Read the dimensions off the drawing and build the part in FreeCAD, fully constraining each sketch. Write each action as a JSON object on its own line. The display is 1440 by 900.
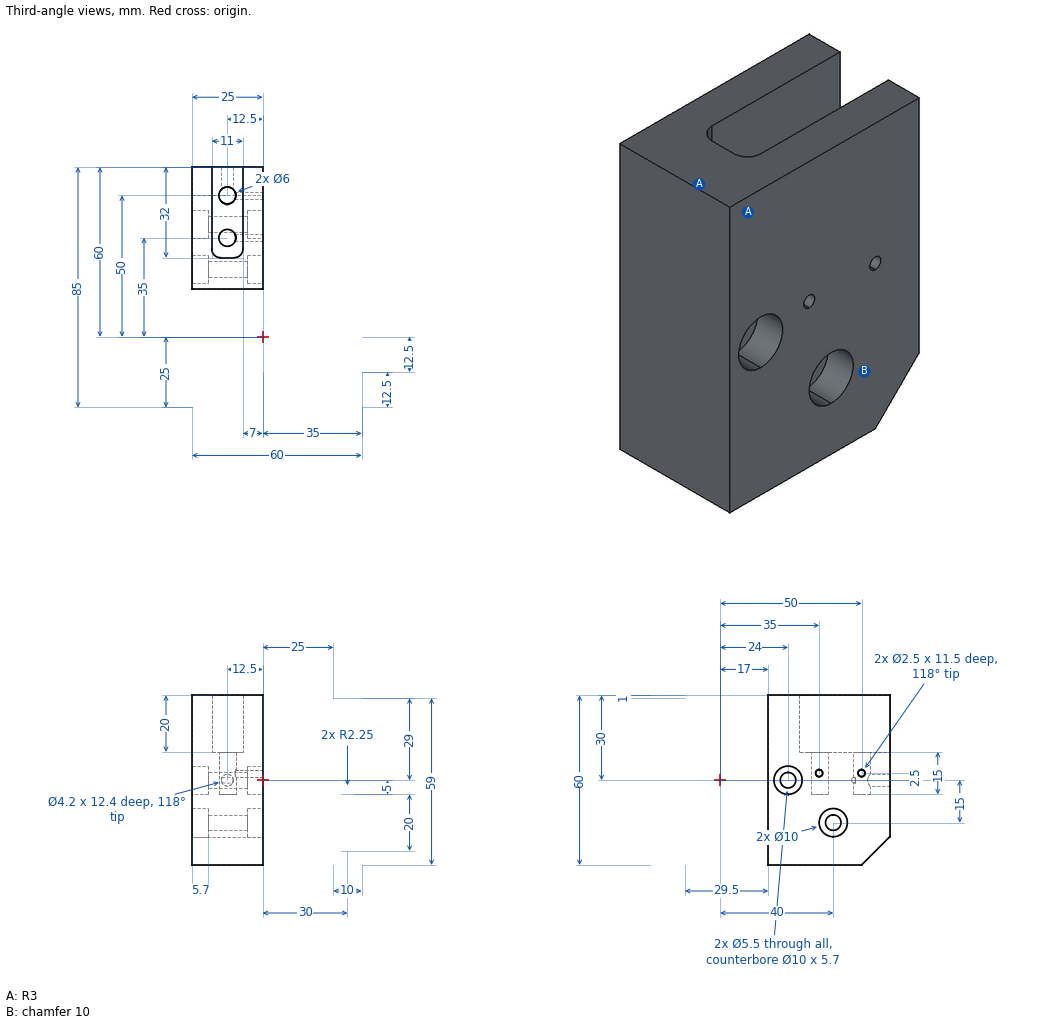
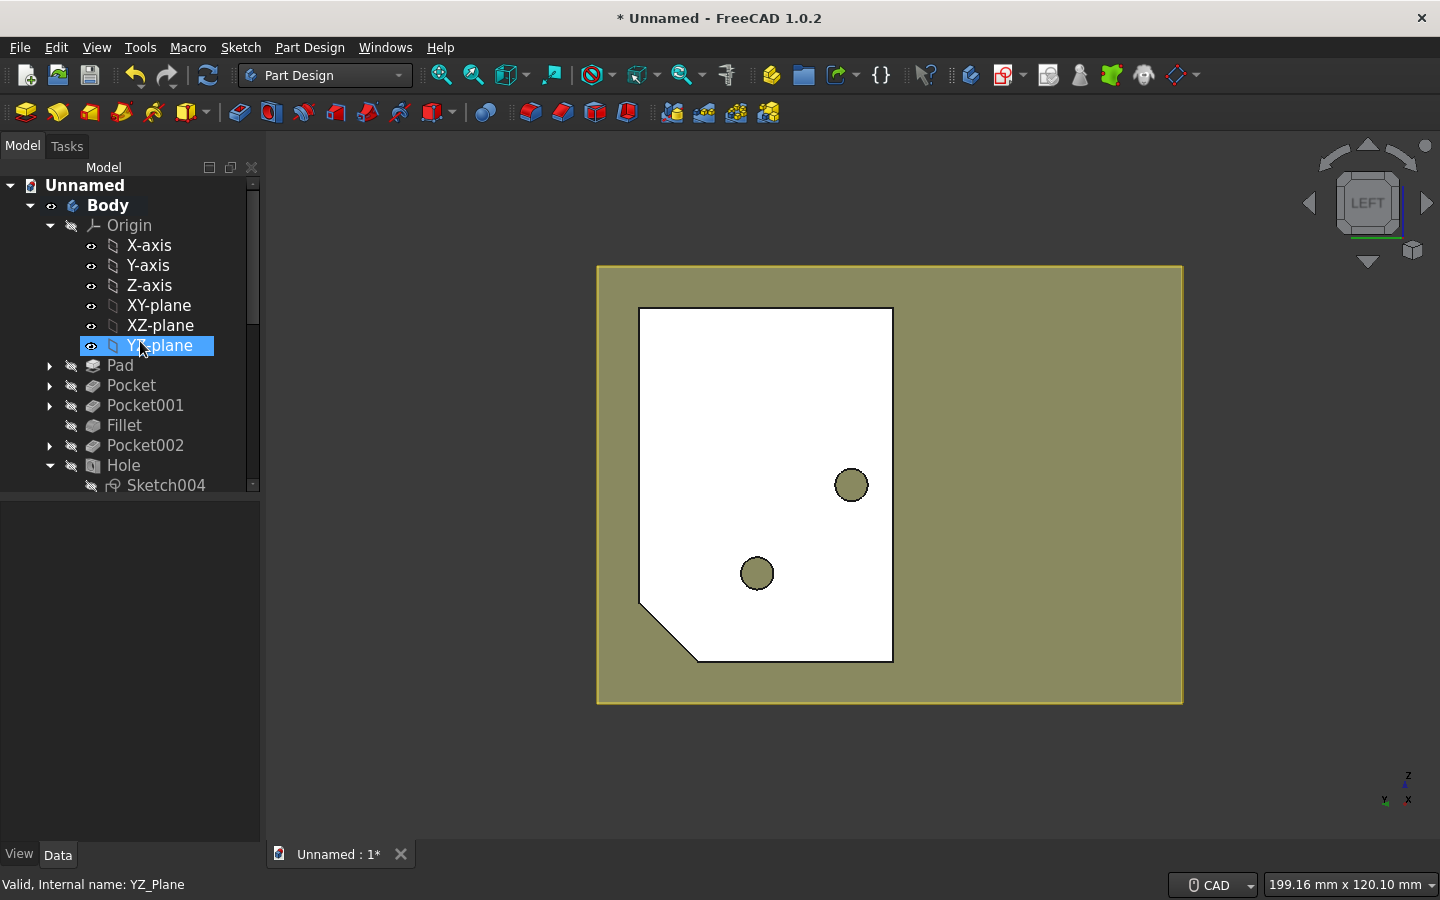
{"action": "scroll", "coordinate": [100, 341], "scroll_direction": "down", "scroll_amount": 6}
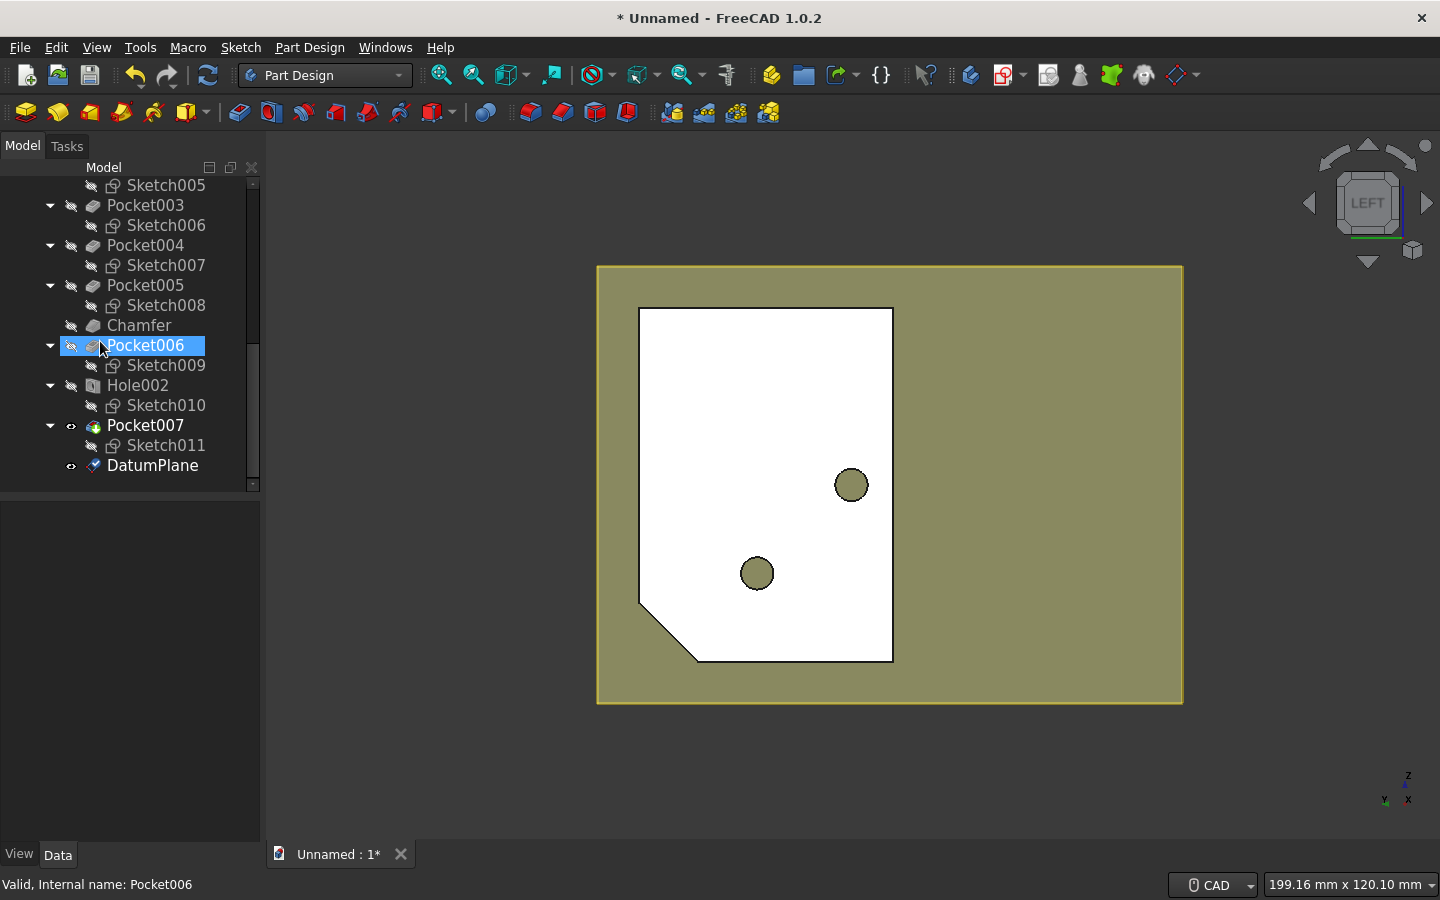
{"action": "left_click", "coordinate": [116, 466]}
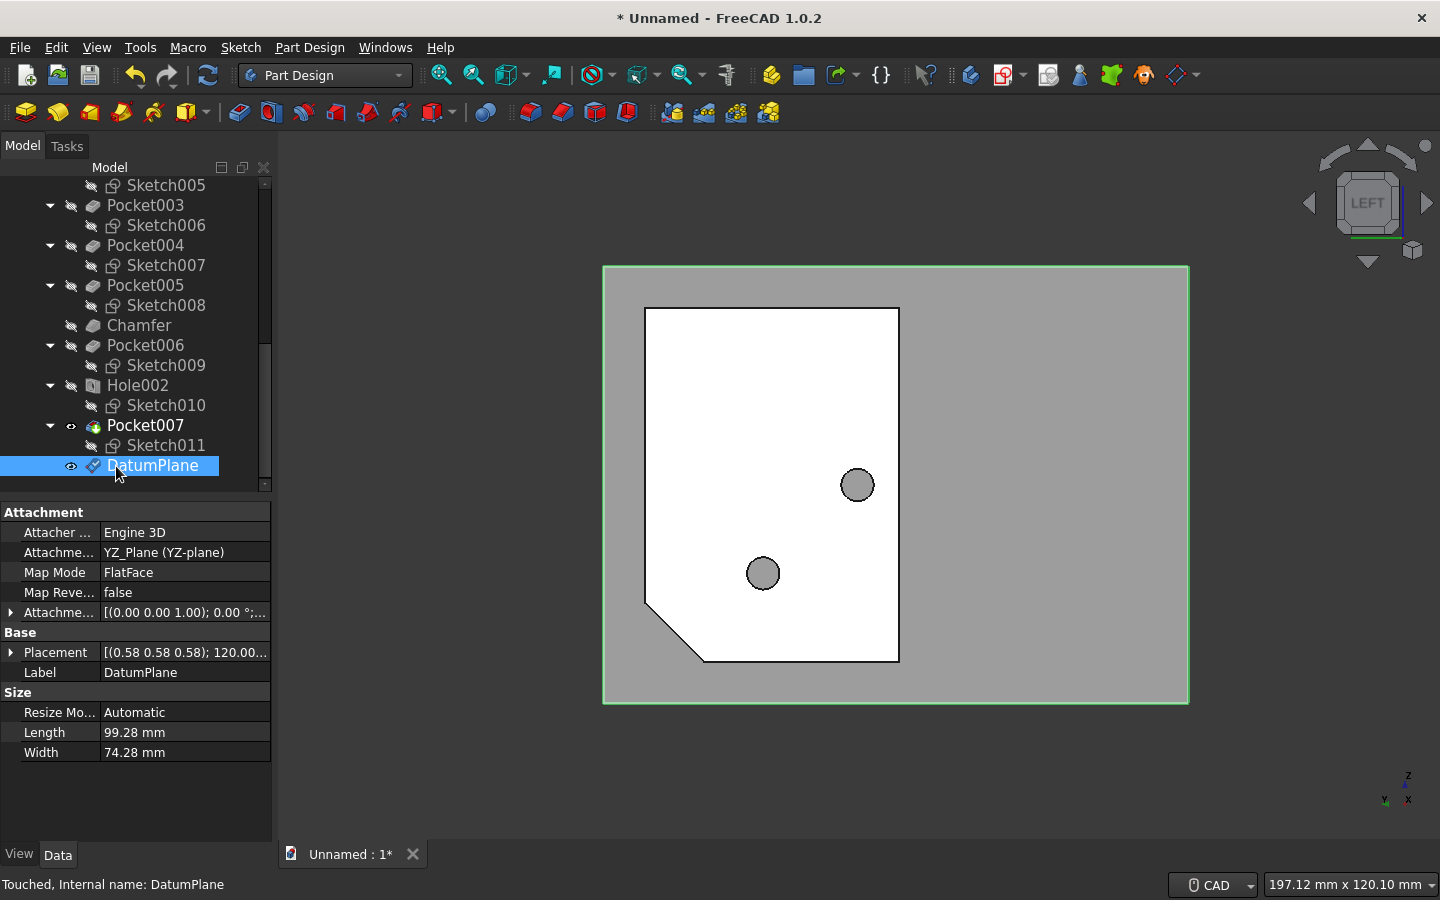
{"action": "left_click", "coordinate": [1004, 76]}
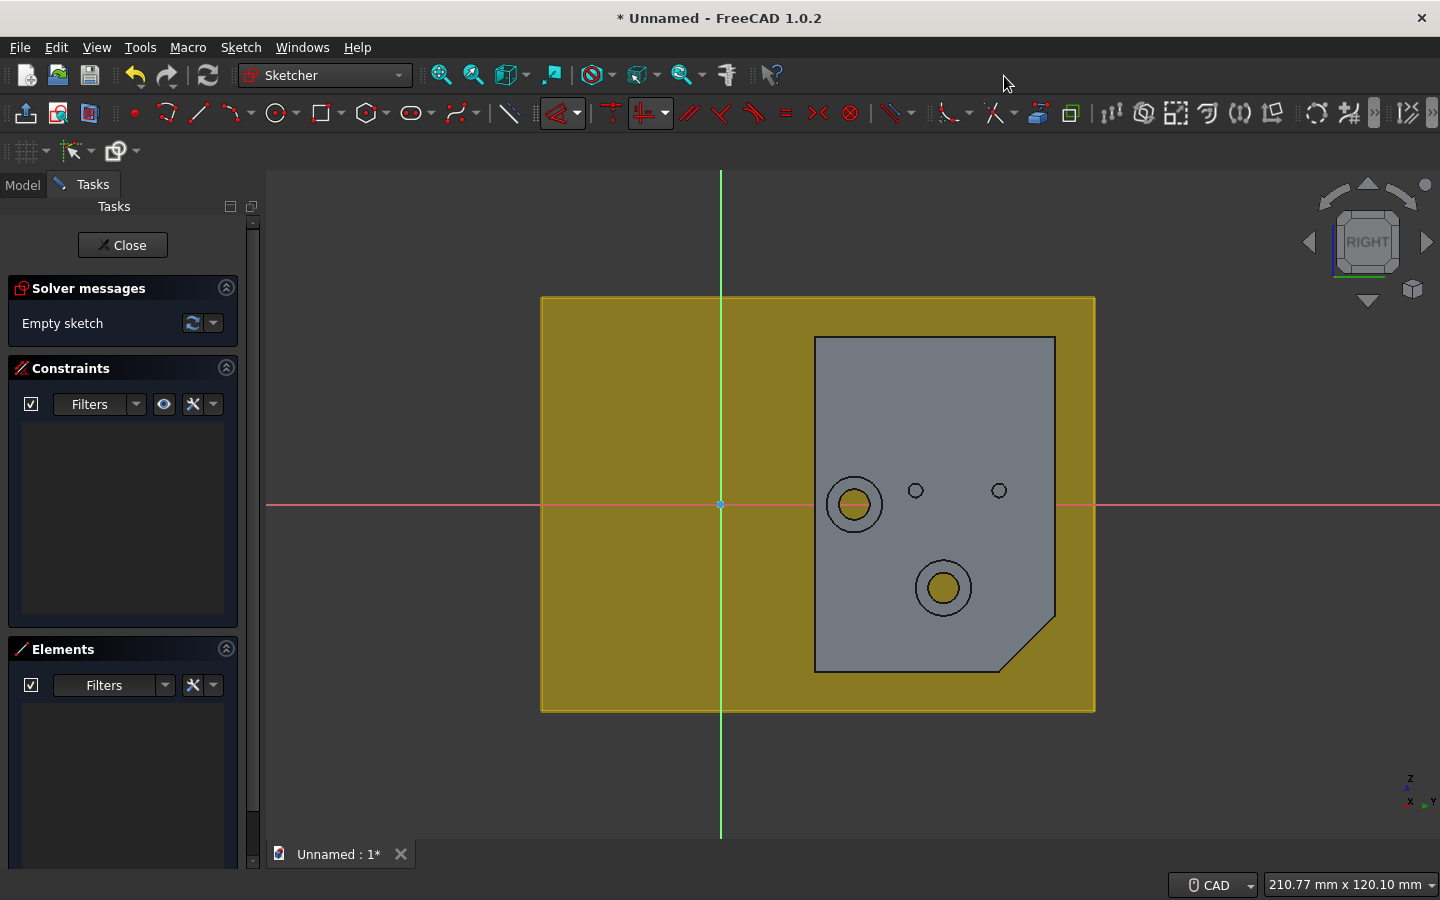
{"action": "left_click", "coordinate": [90, 114]}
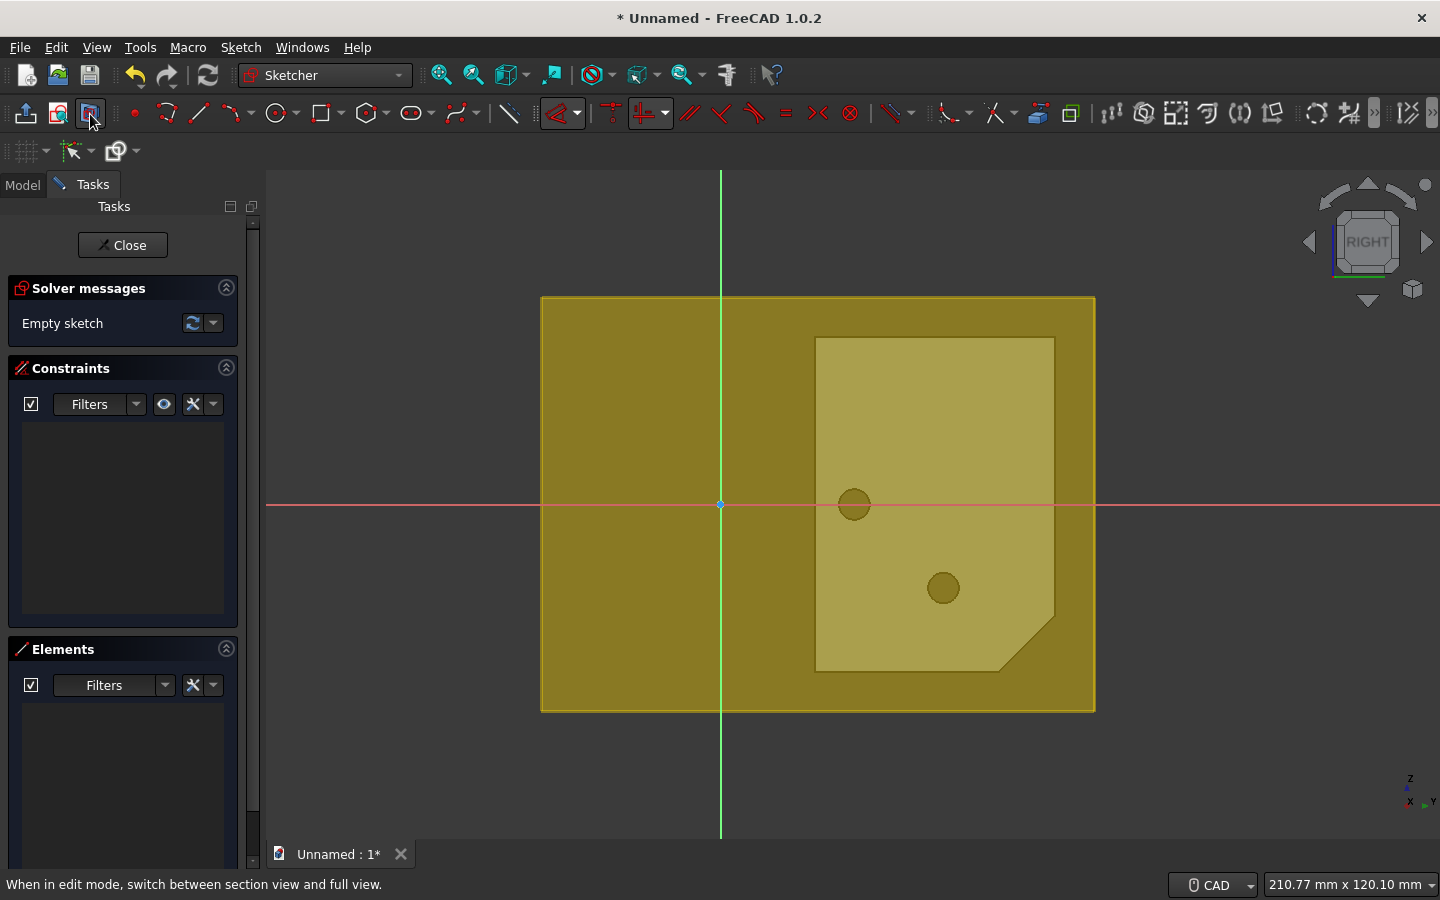
{"action": "scroll", "coordinate": [882, 571], "scroll_direction": "up", "scroll_amount": 5}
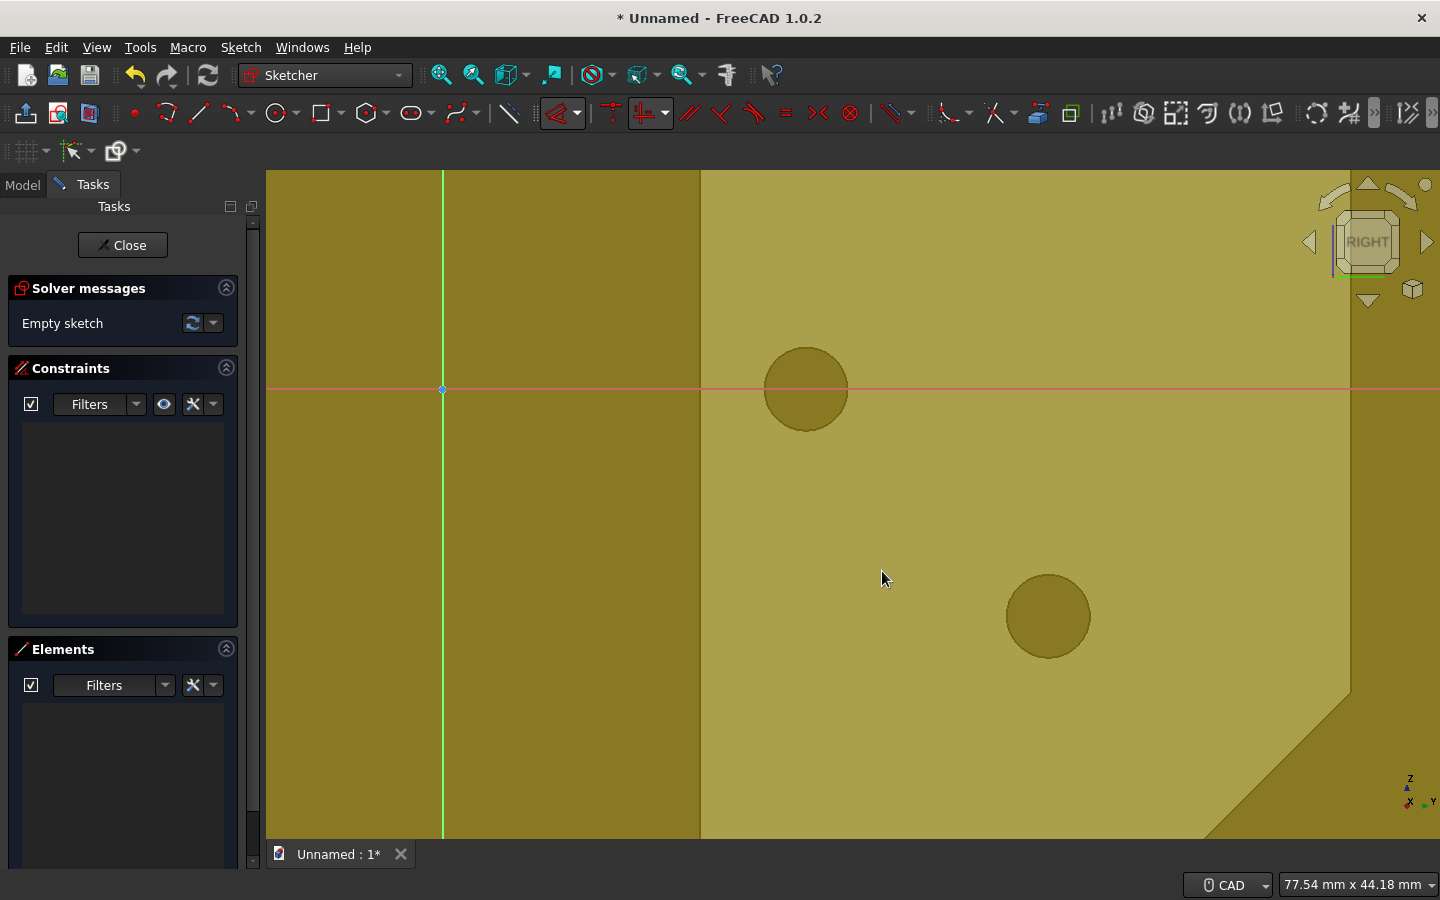
{"action": "left_click", "coordinate": [276, 114]}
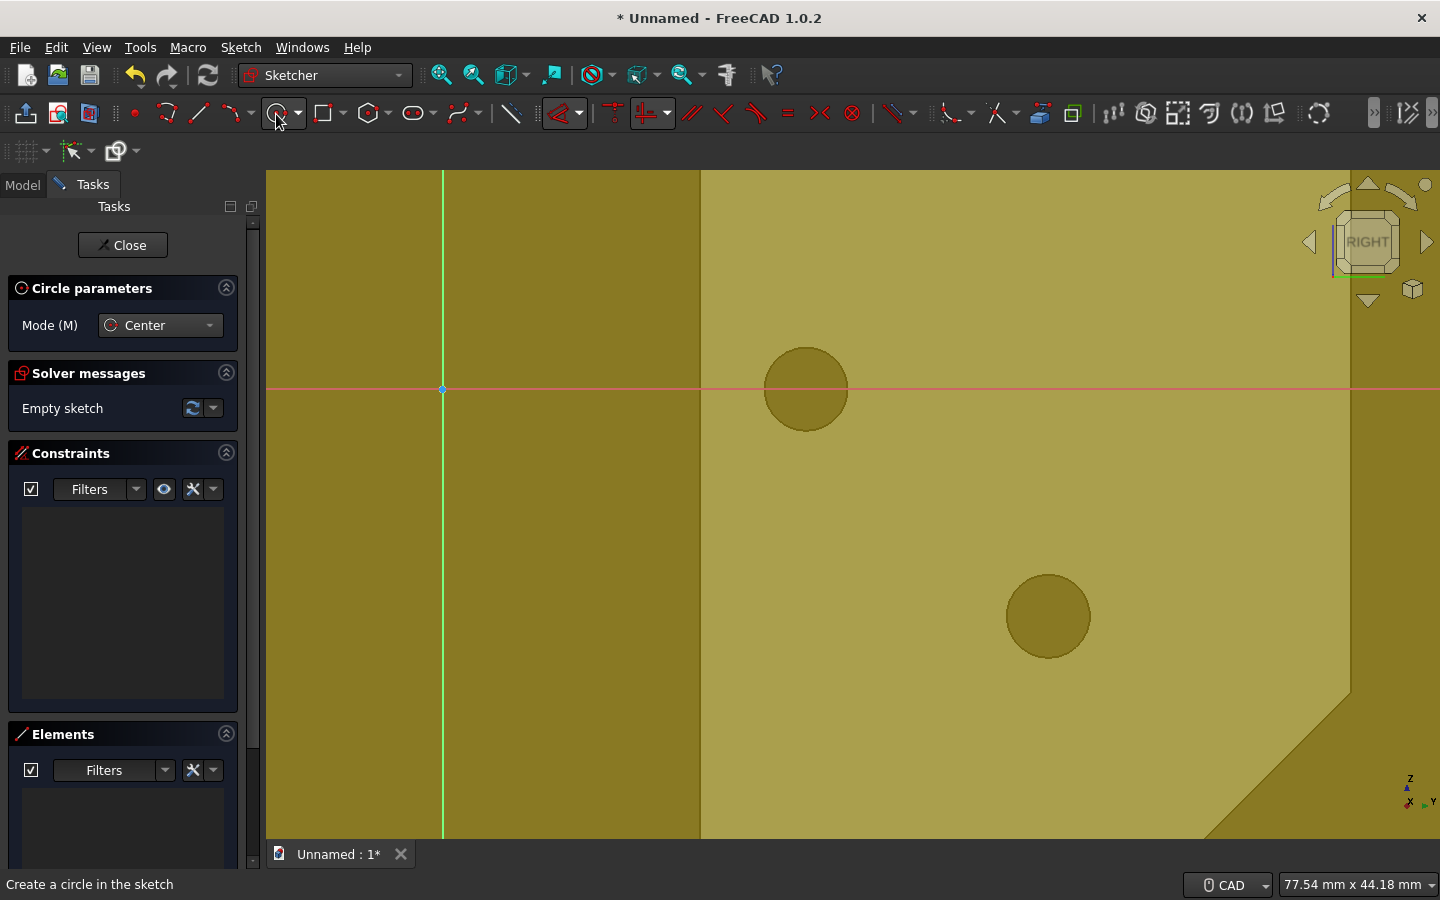
{"action": "left_click", "coordinate": [1048, 616]}
{"action": "mouse_move", "coordinate": [1102, 563]}